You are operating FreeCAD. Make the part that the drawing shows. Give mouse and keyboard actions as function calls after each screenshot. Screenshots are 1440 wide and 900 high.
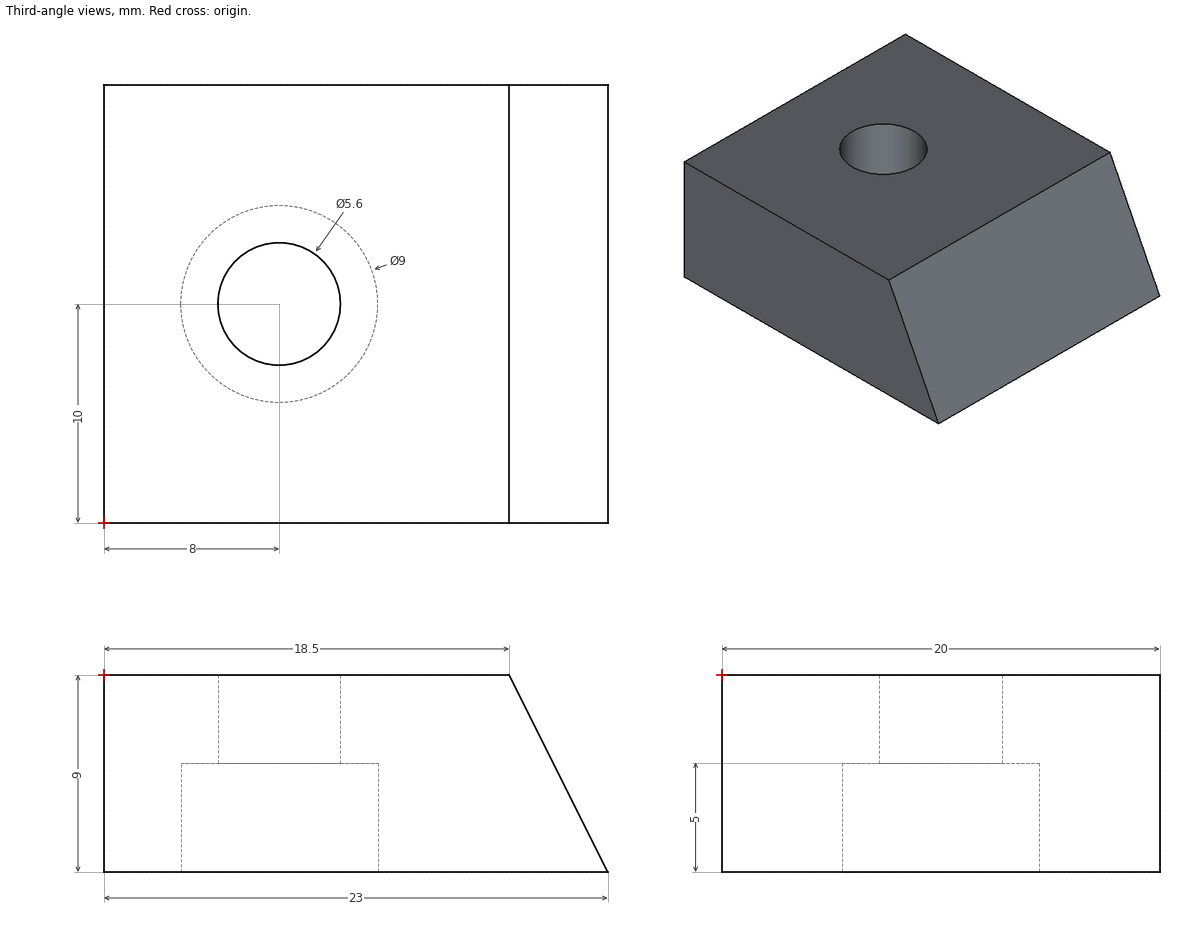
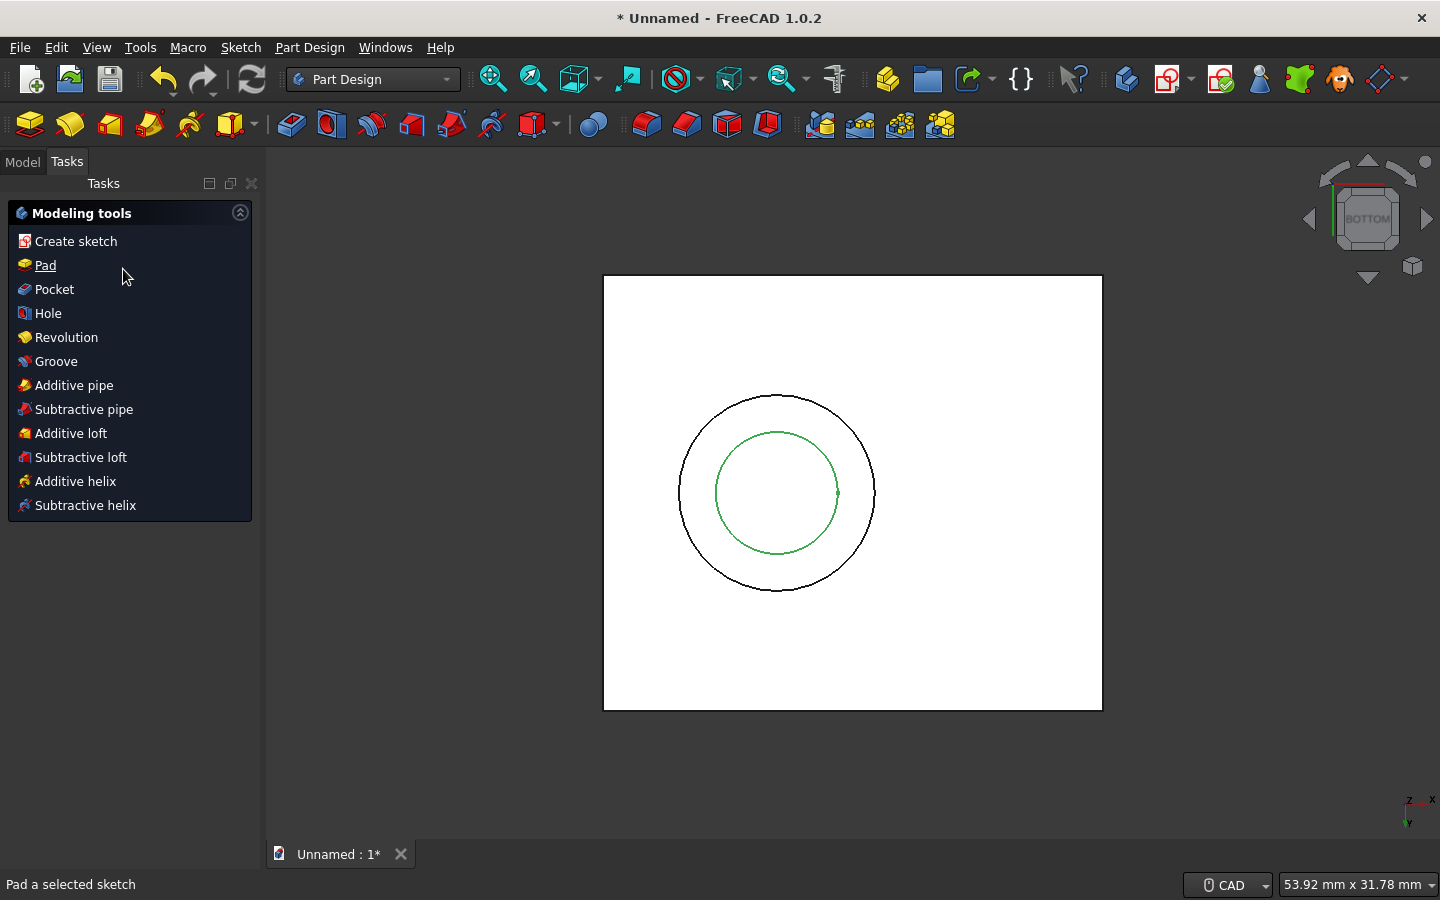
click(292, 124)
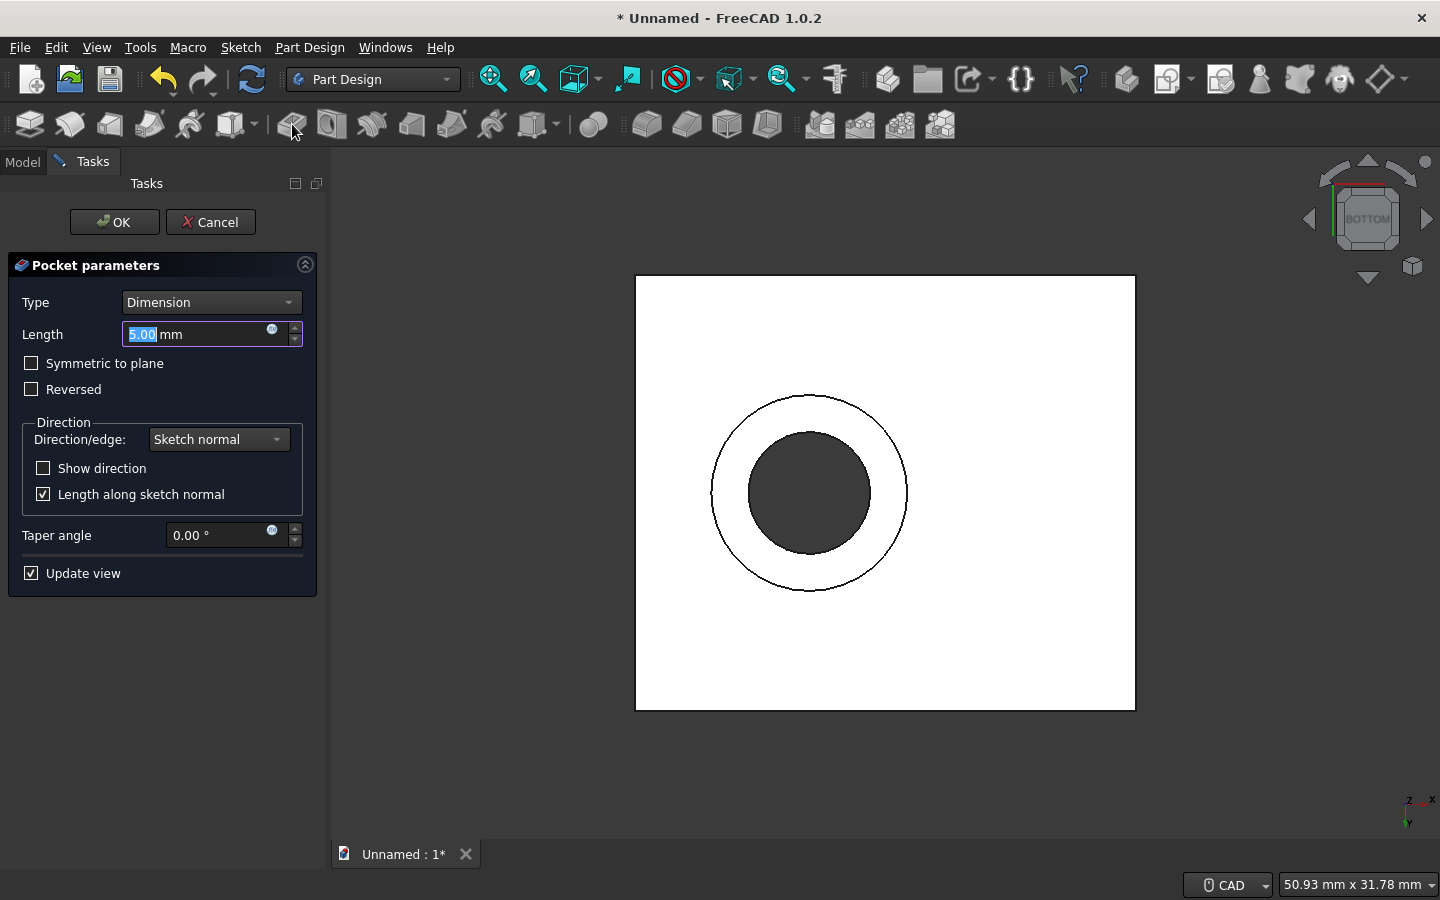
click(212, 302)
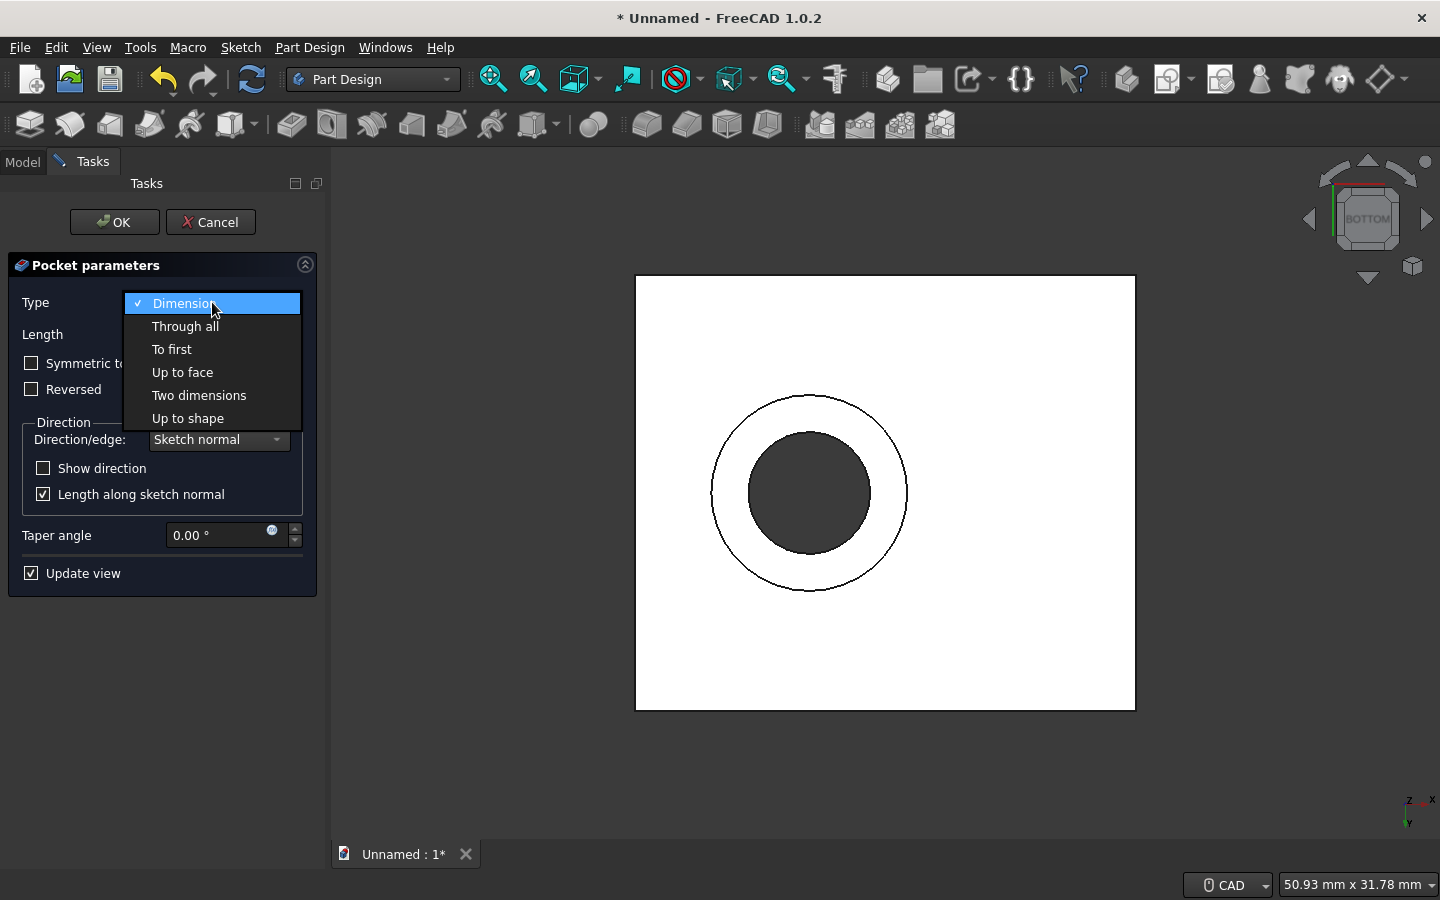
click(212, 326)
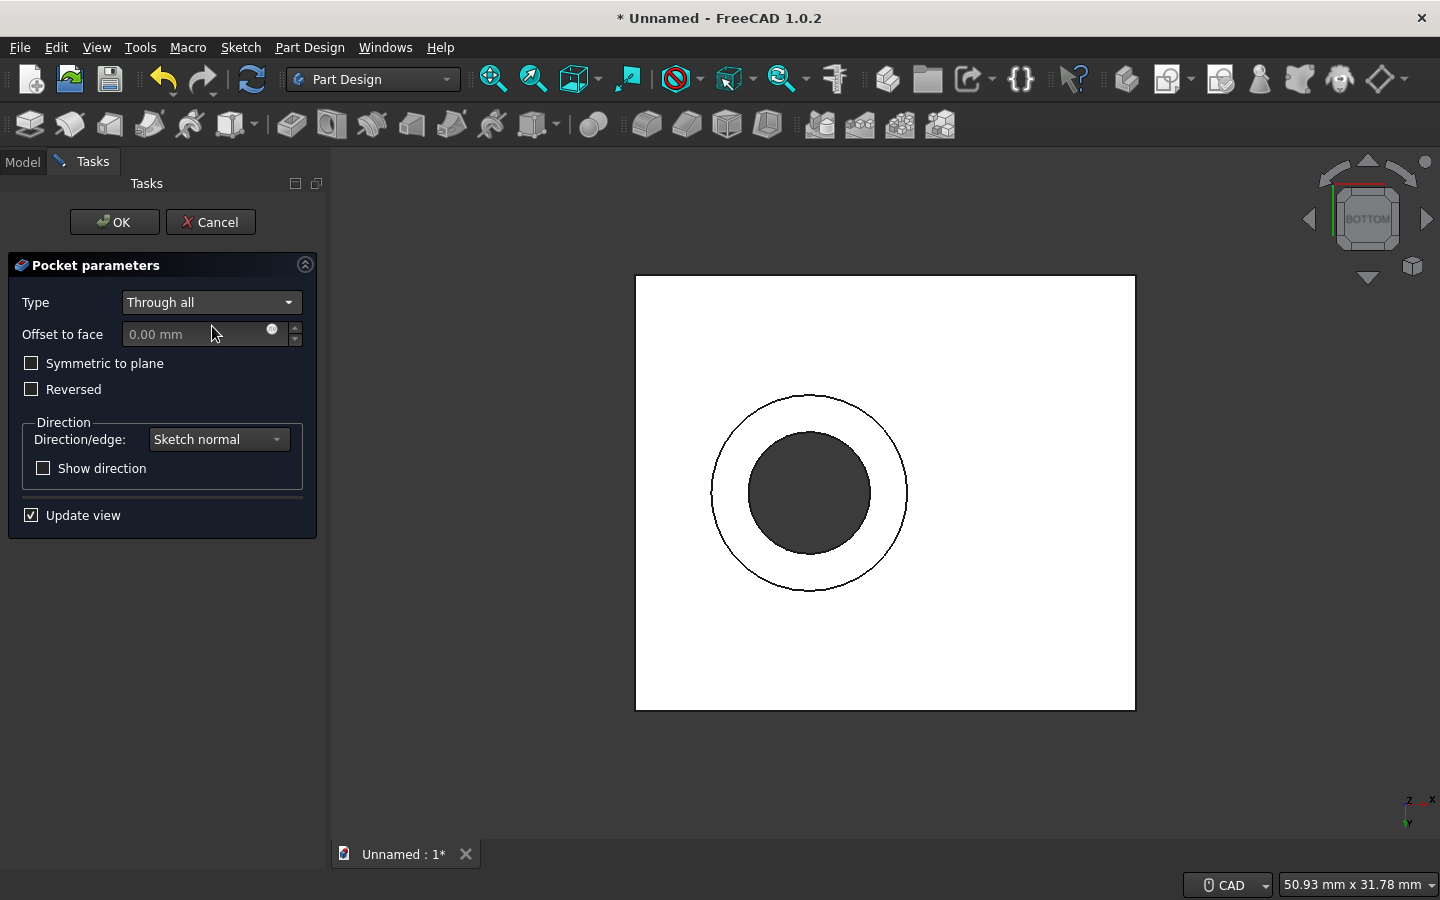
click(115, 222)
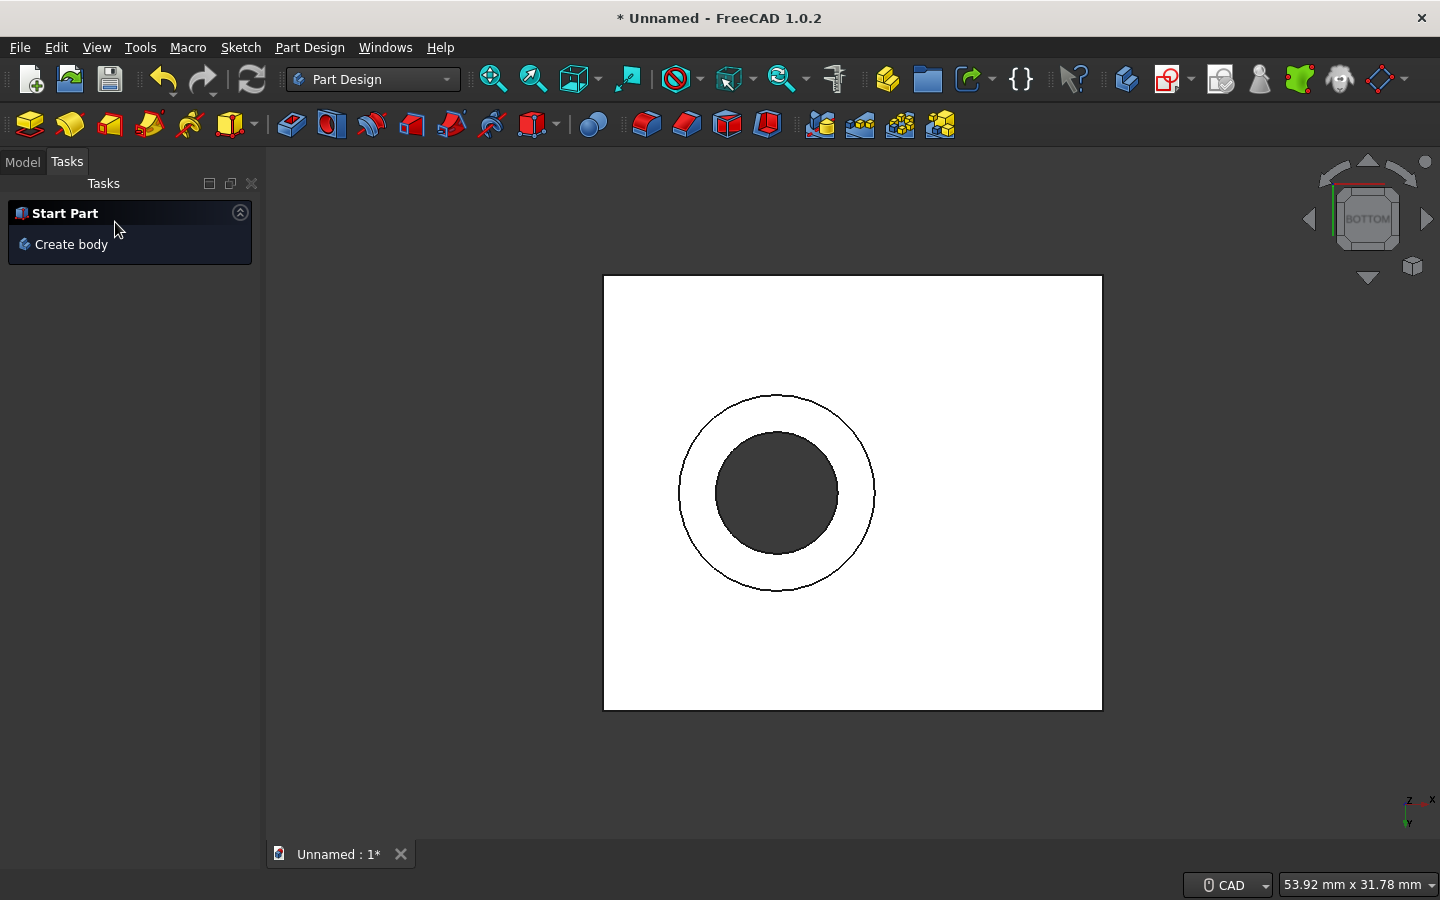
key(0)